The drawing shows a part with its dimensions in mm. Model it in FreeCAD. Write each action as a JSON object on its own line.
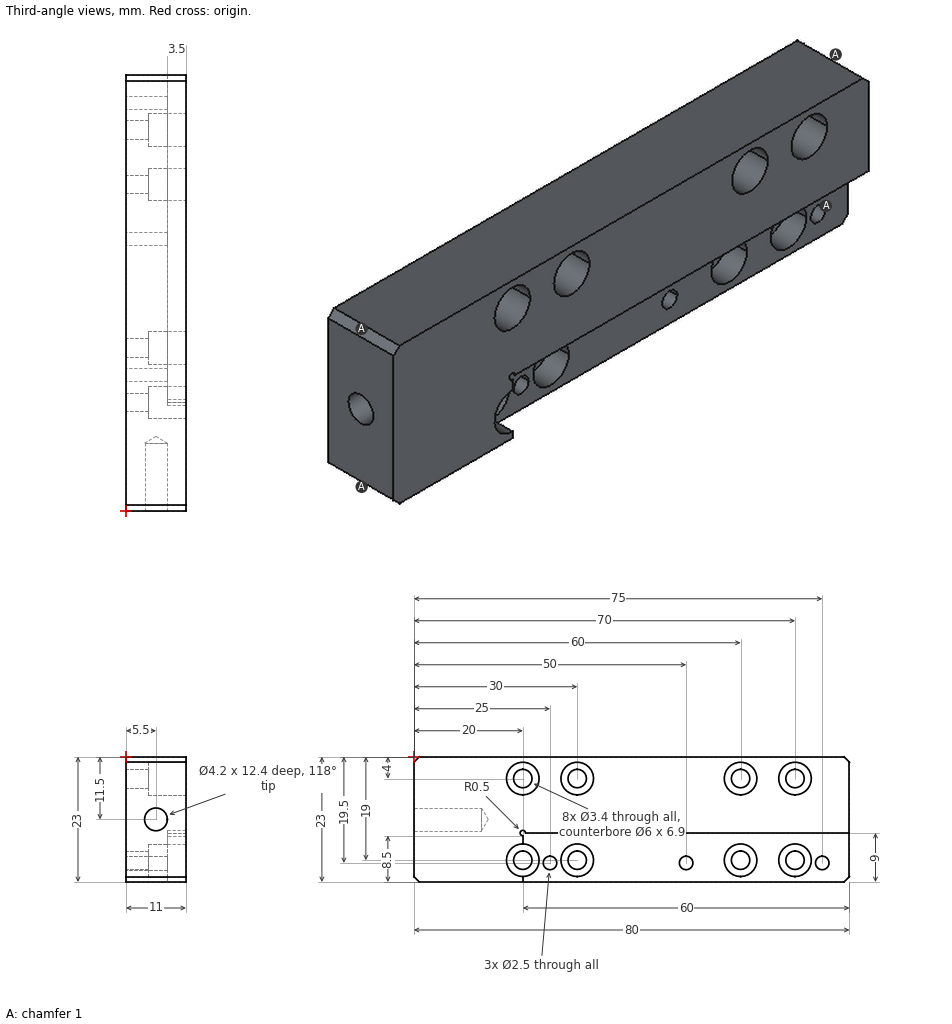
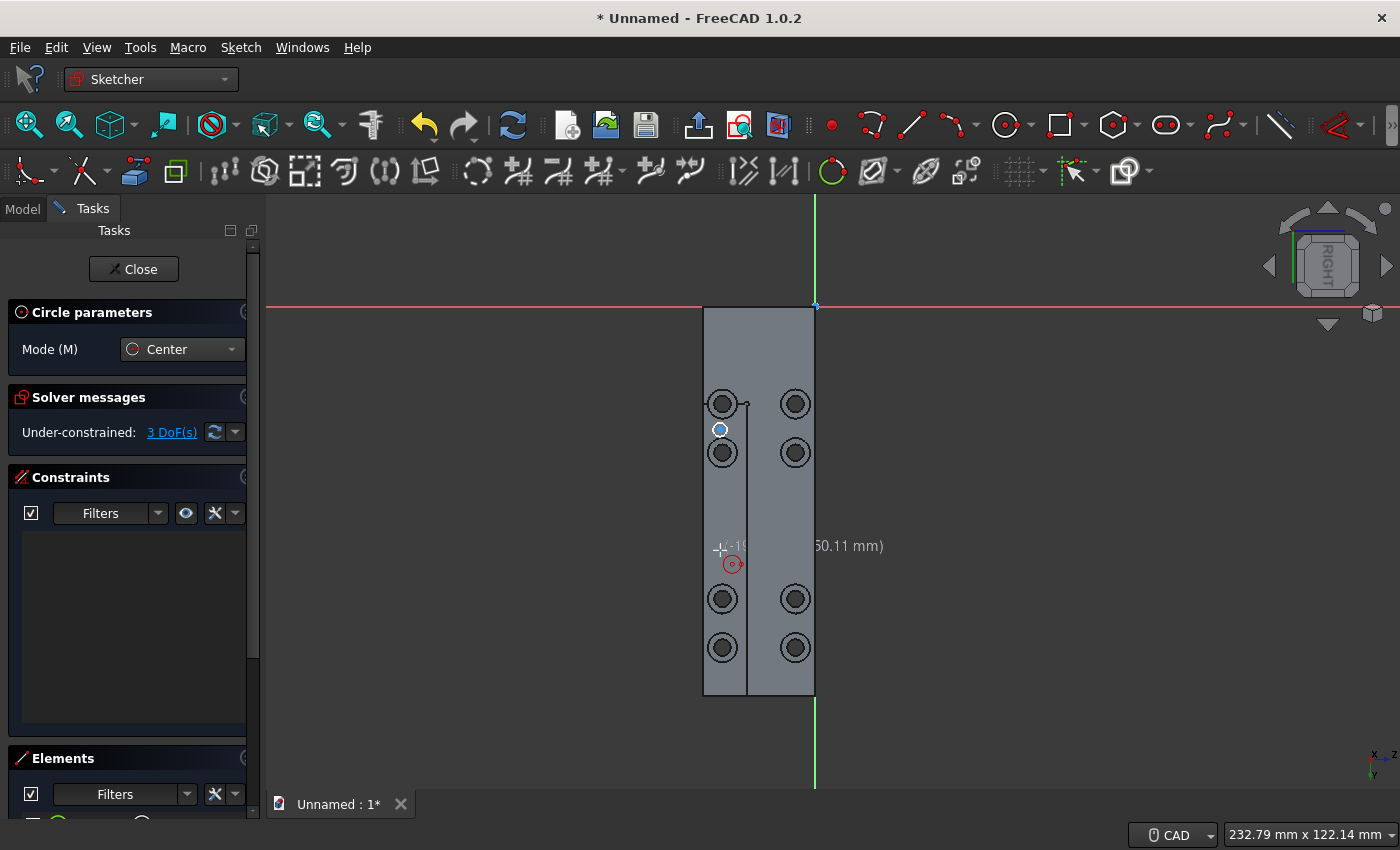
{"action": "left_click", "coordinate": [720, 550]}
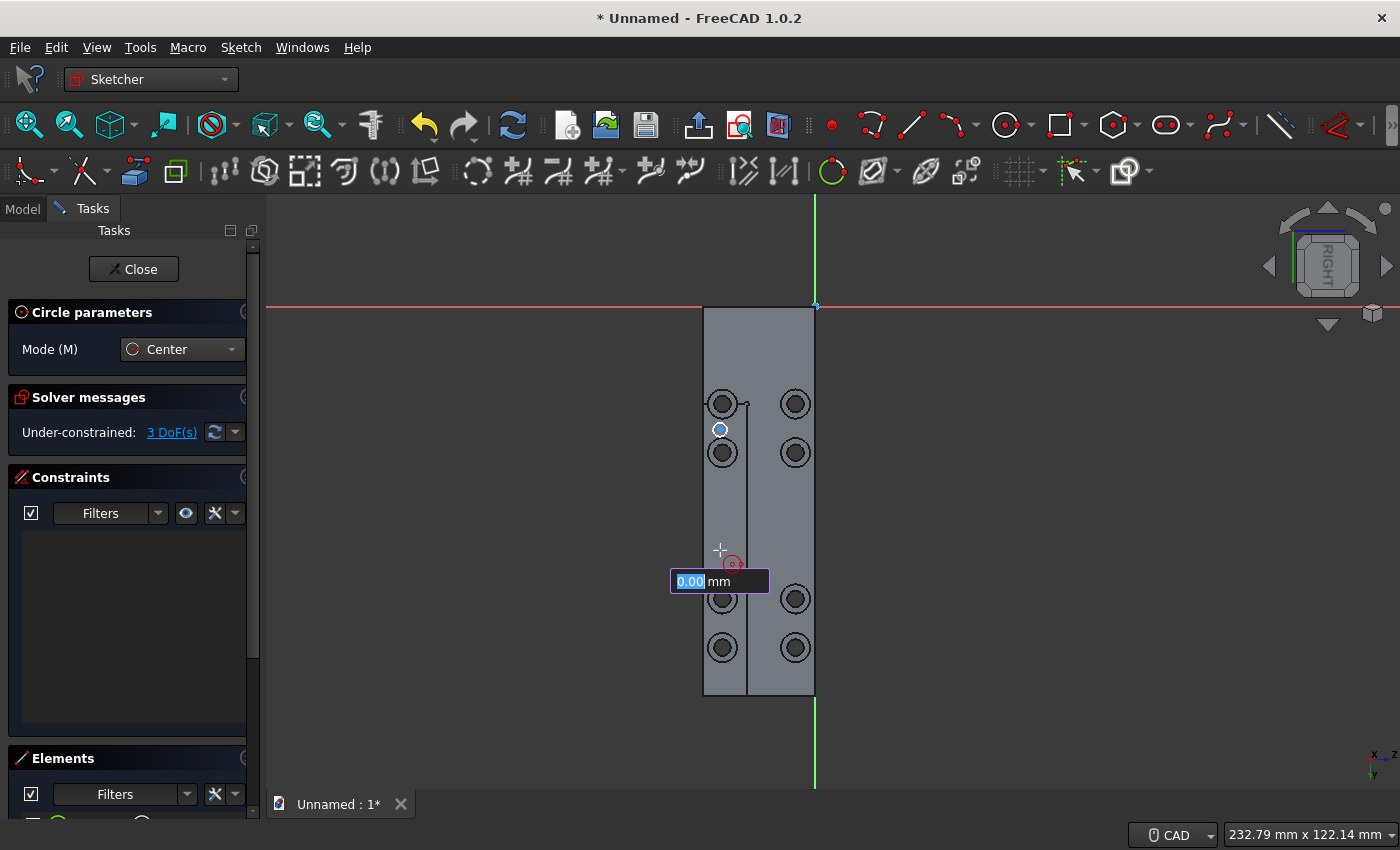
{"action": "scroll", "coordinate": [724, 546], "scroll_direction": "up", "scroll_amount": 5}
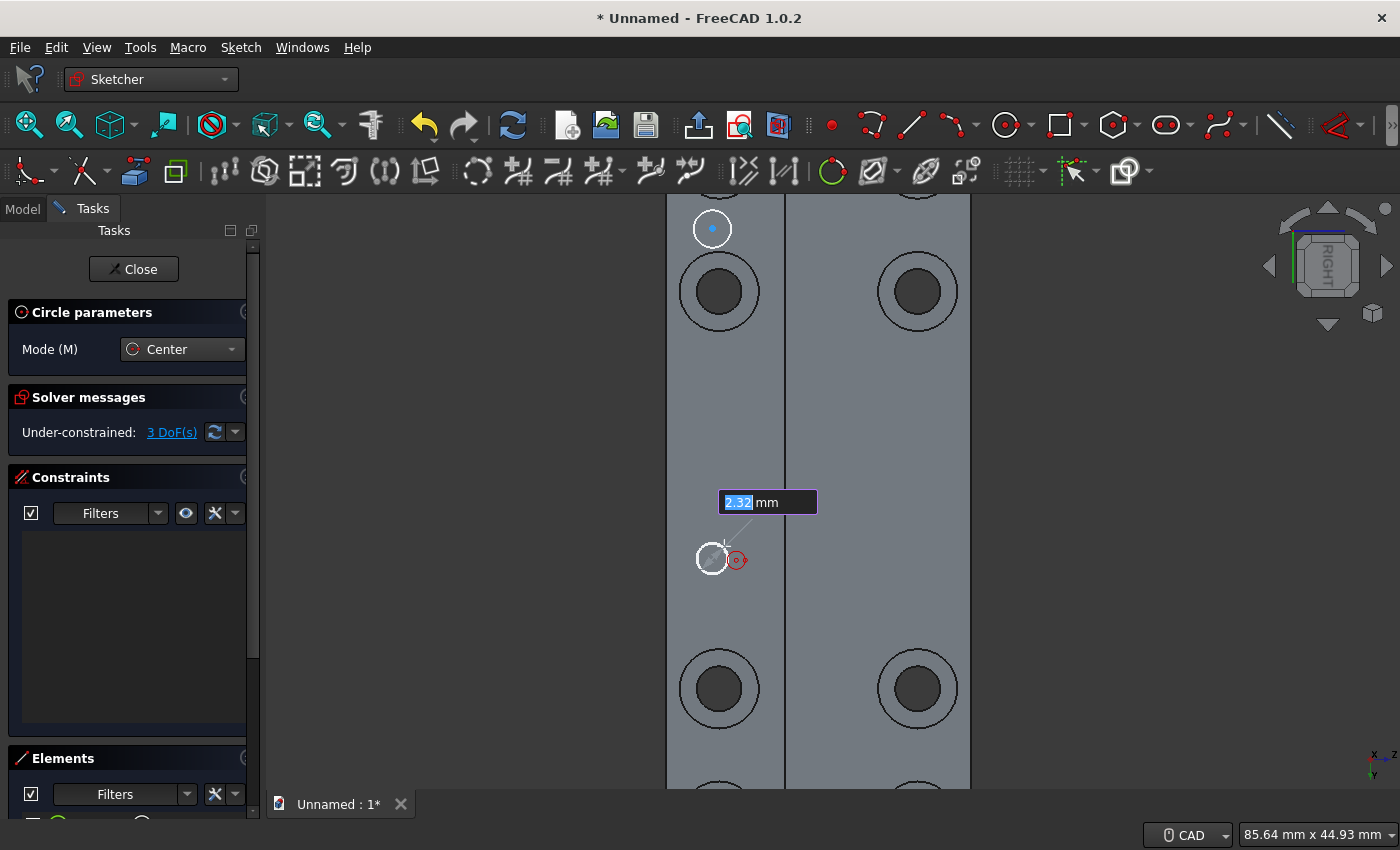
{"action": "left_click", "coordinate": [724, 545]}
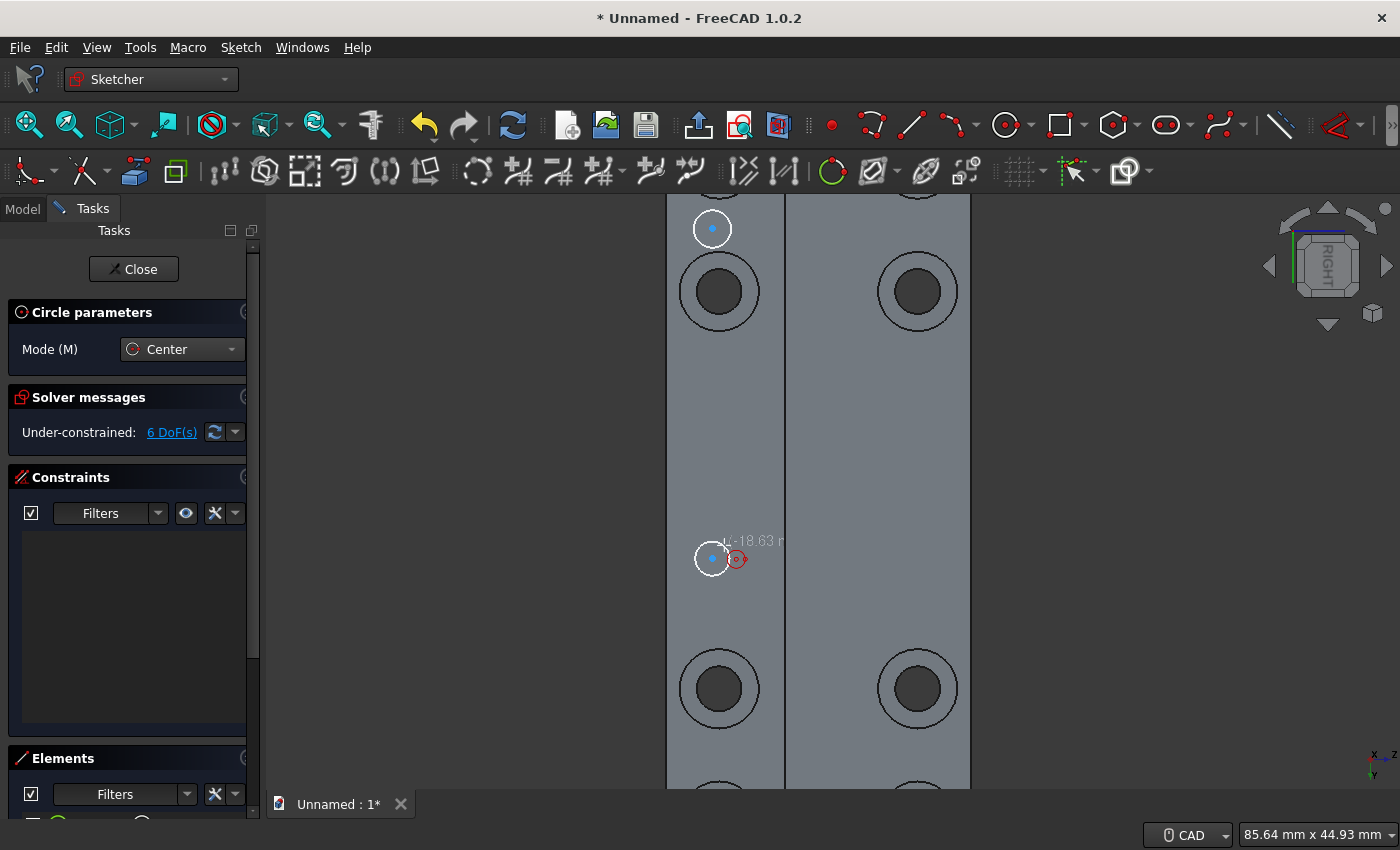
{"action": "scroll", "coordinate": [724, 545], "scroll_direction": "down", "scroll_amount": 5}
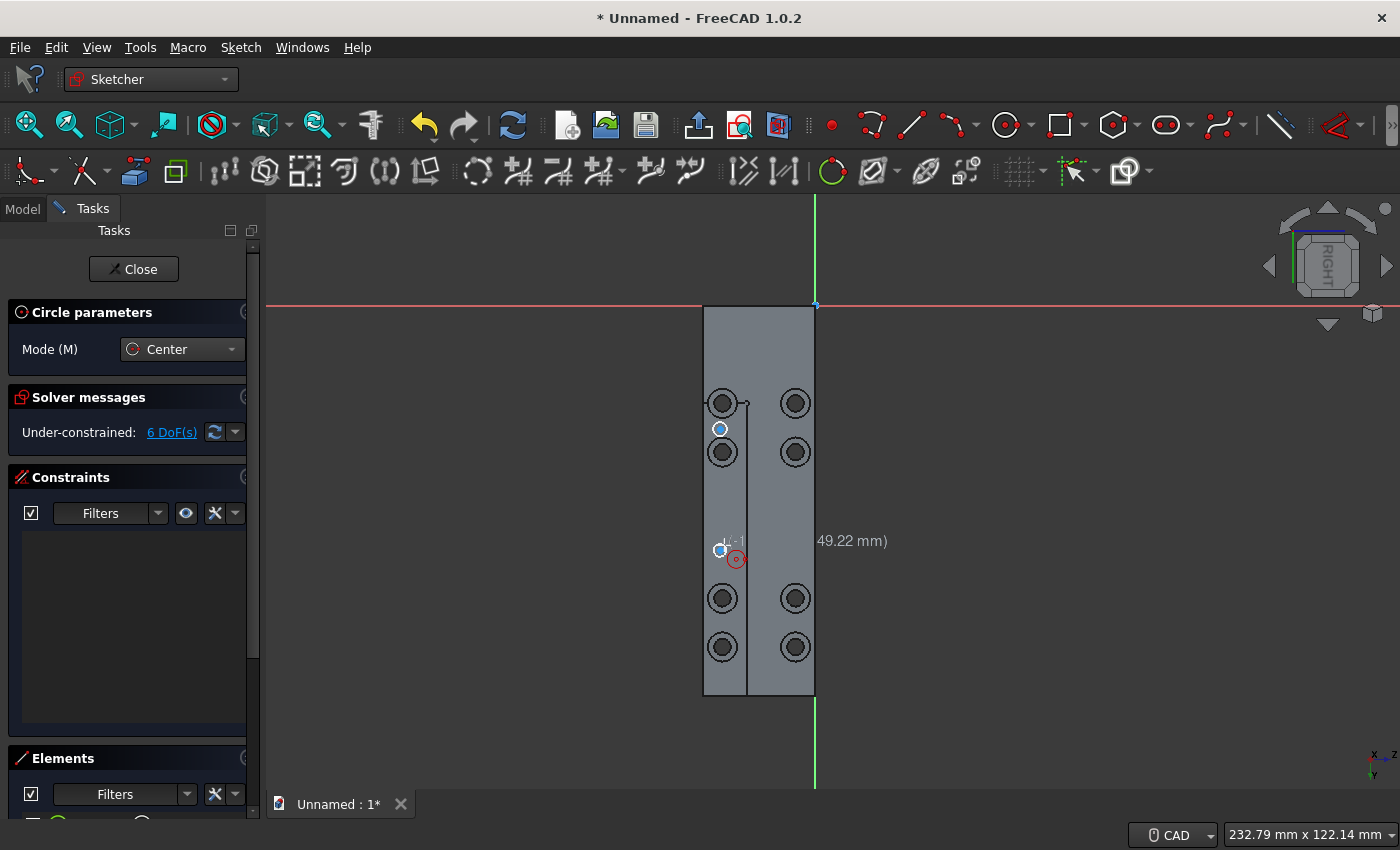
{"action": "scroll", "coordinate": [720, 671], "scroll_direction": "up", "scroll_amount": 7}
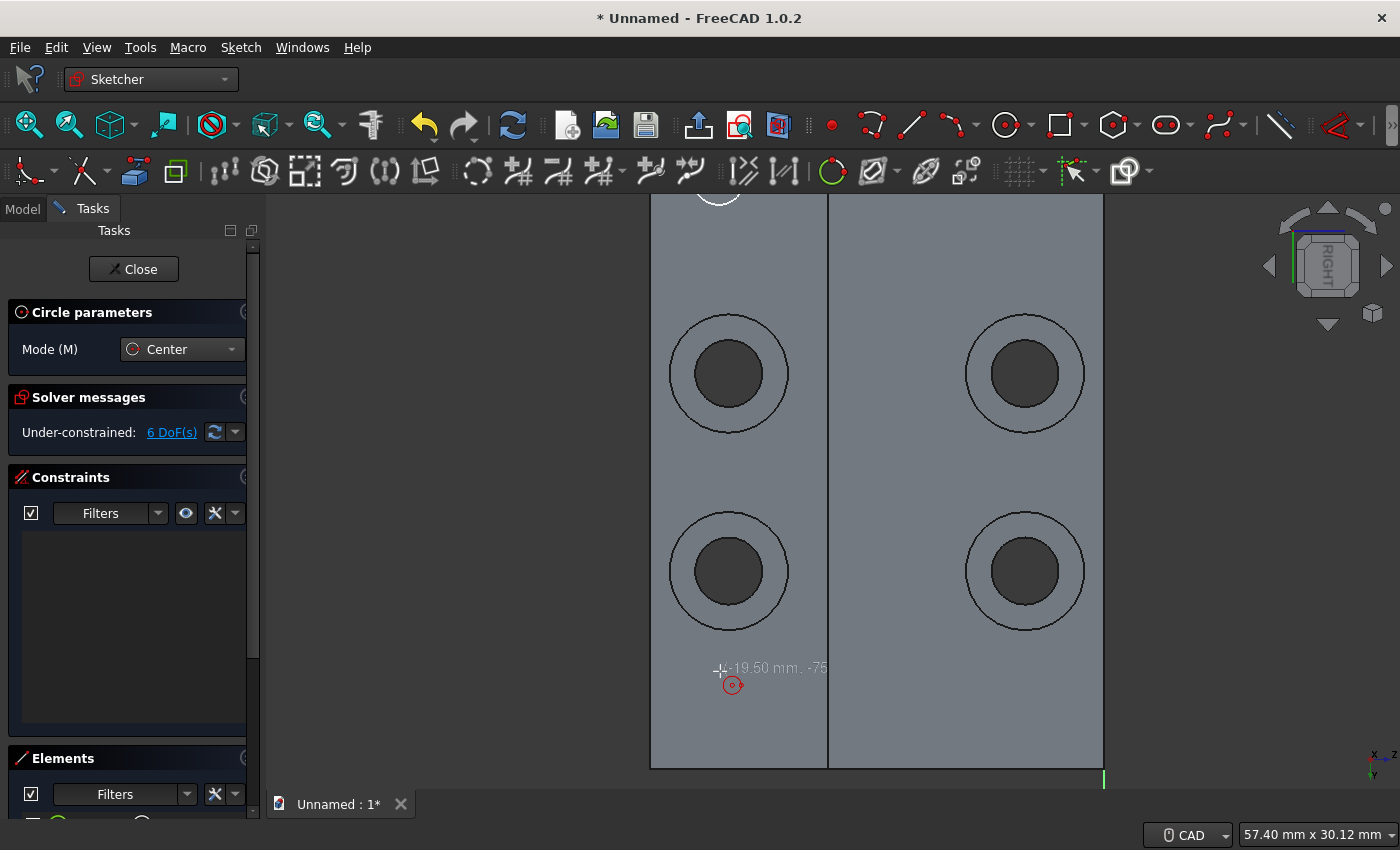
{"action": "scroll", "coordinate": [720, 672], "scroll_direction": "down", "scroll_amount": 7}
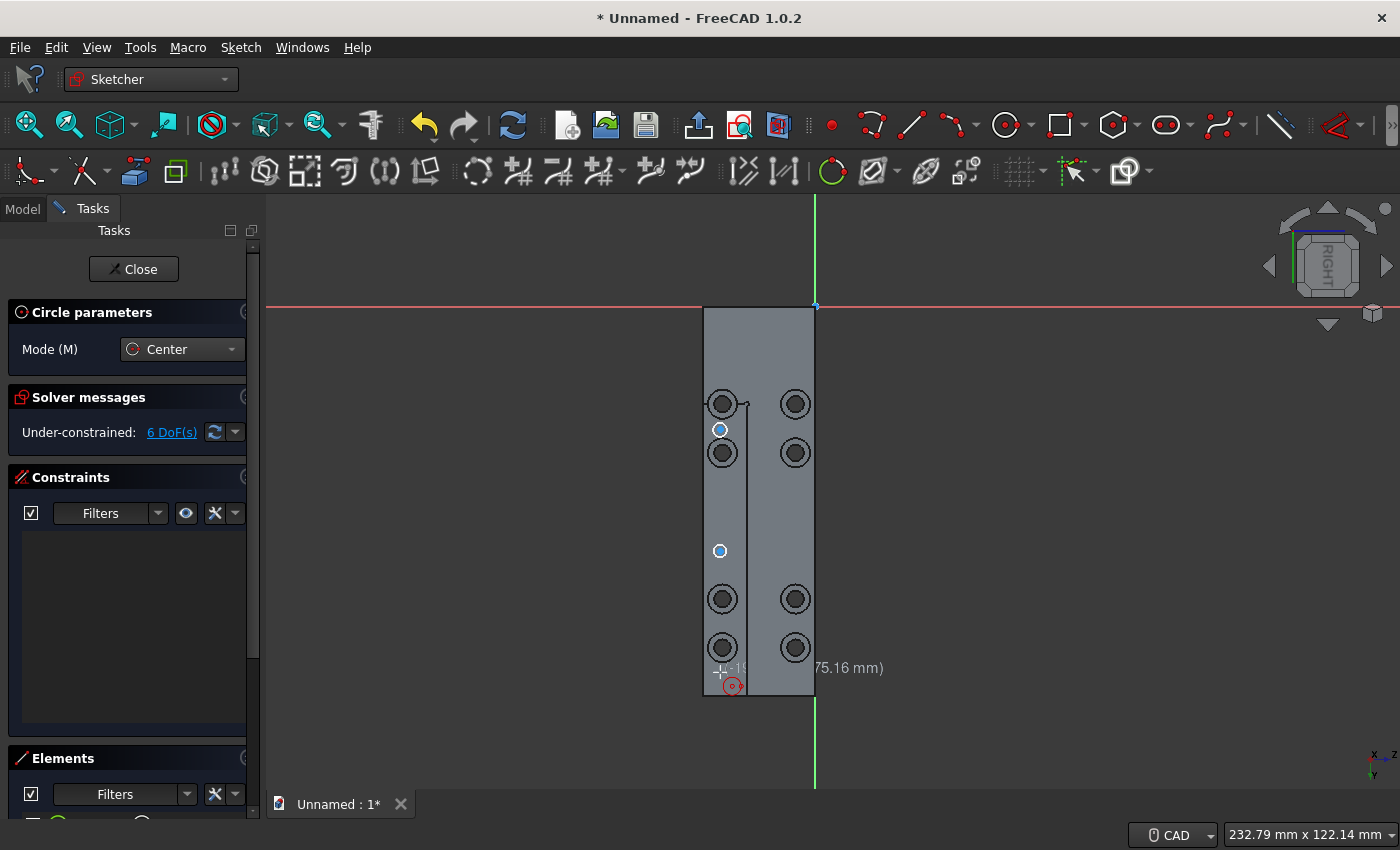
{"action": "left_click", "coordinate": [720, 672]}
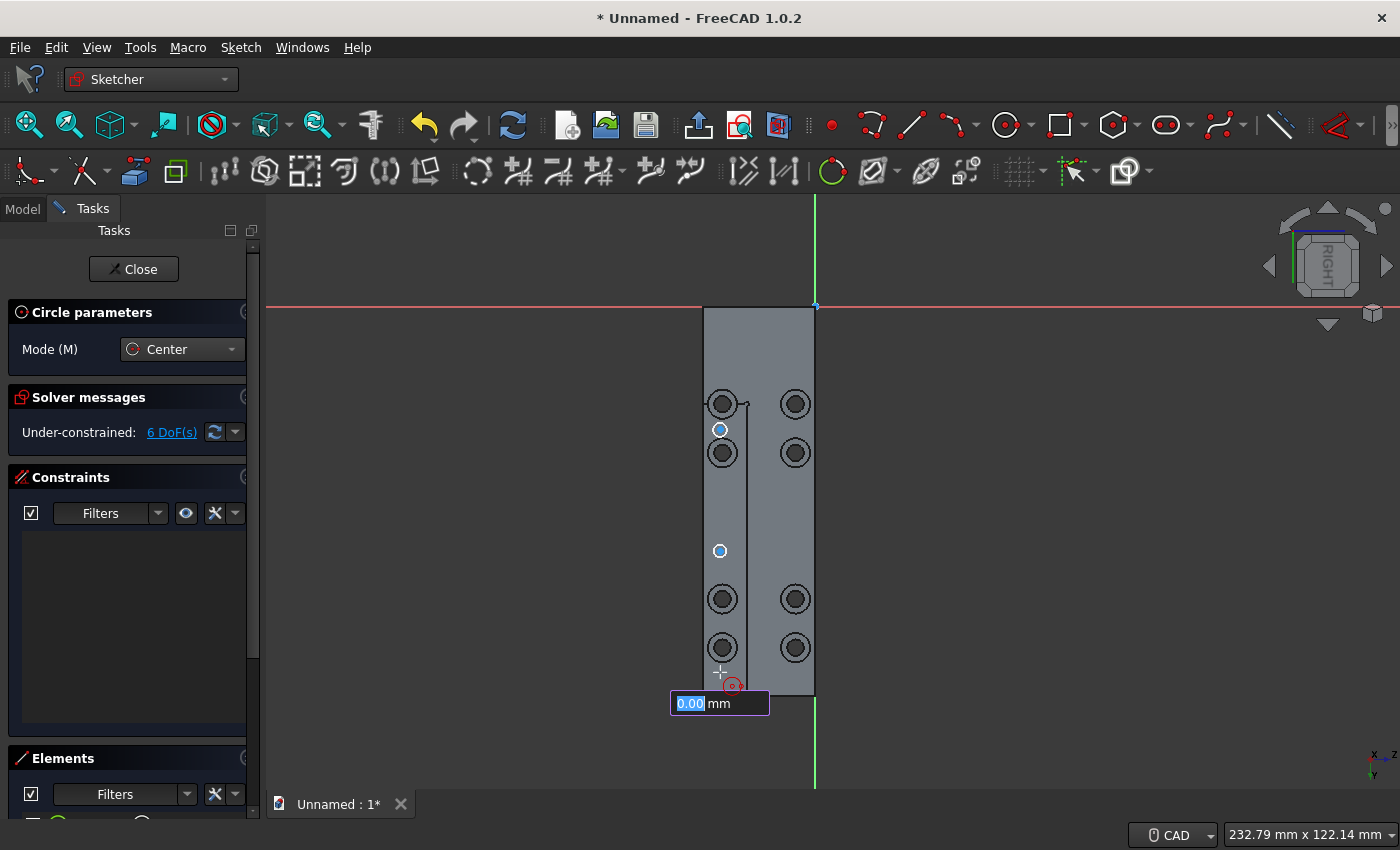
{"action": "scroll", "coordinate": [724, 668], "scroll_direction": "up", "scroll_amount": 5}